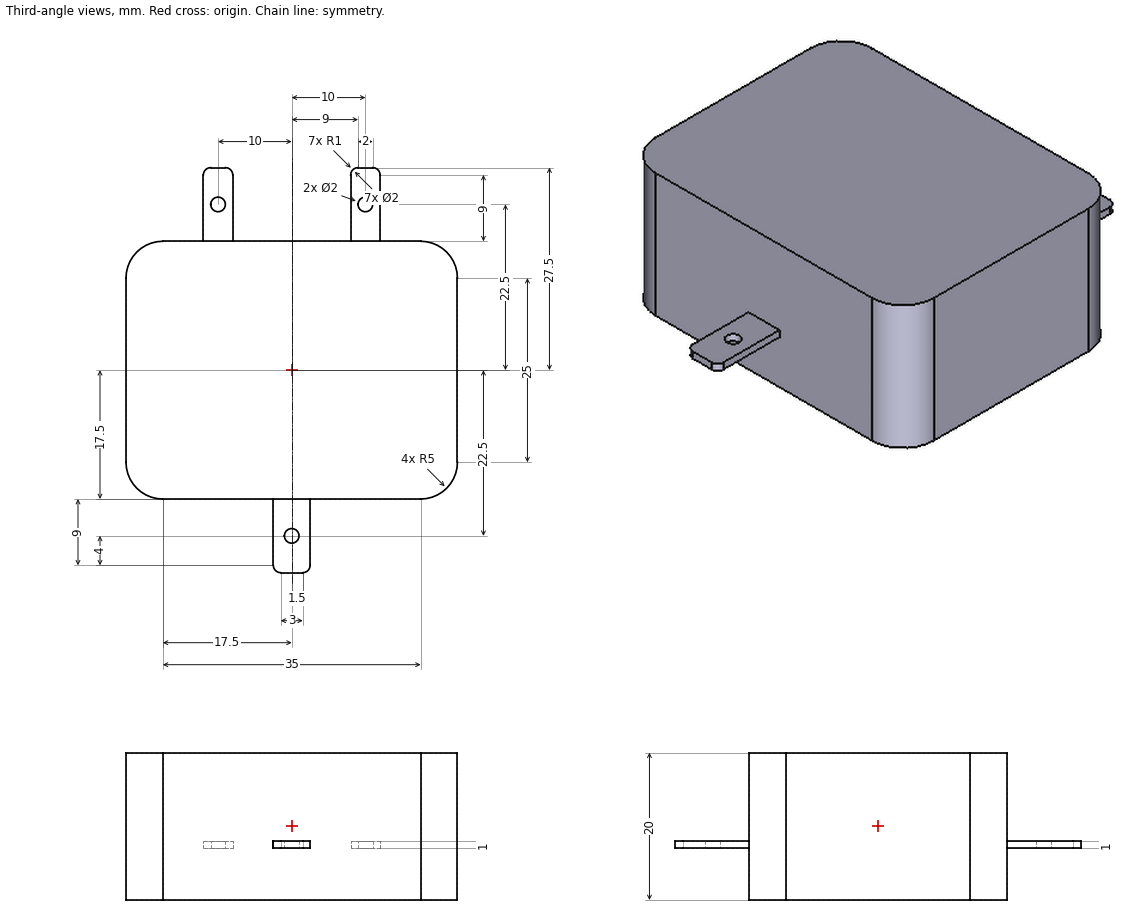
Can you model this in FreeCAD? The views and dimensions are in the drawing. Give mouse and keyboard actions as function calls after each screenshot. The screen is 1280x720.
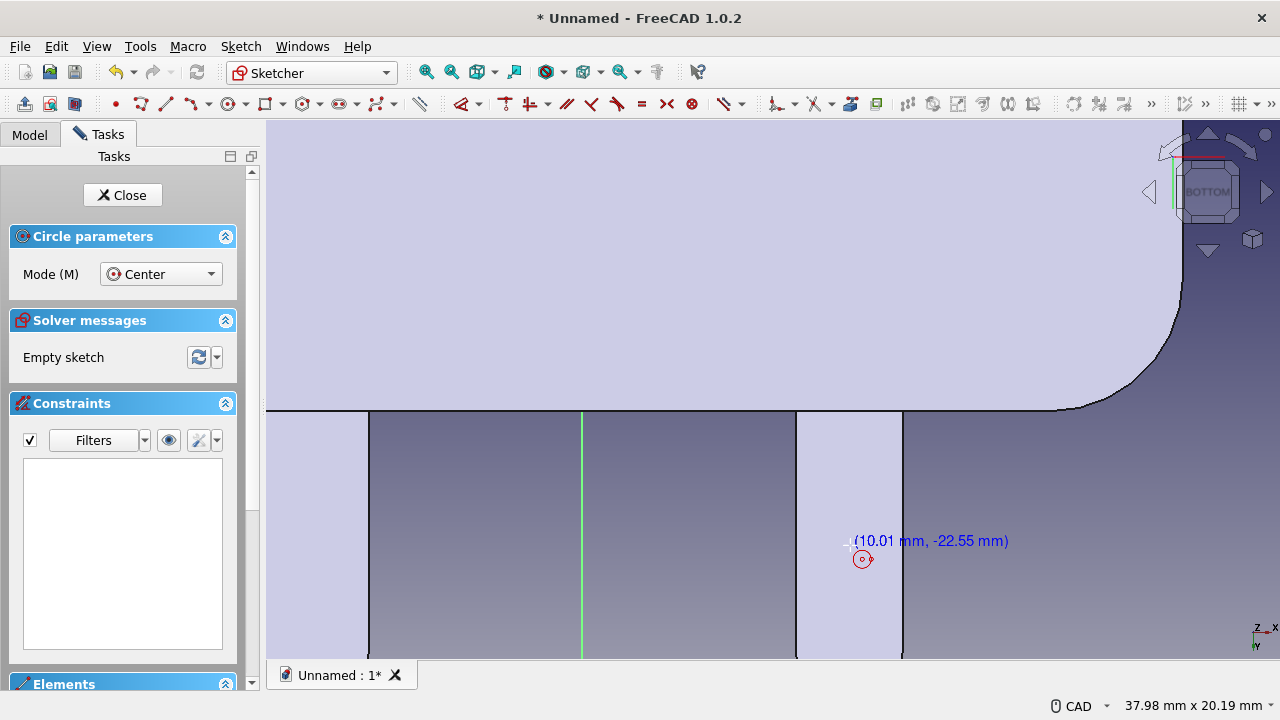
click(849, 545)
click(868, 526)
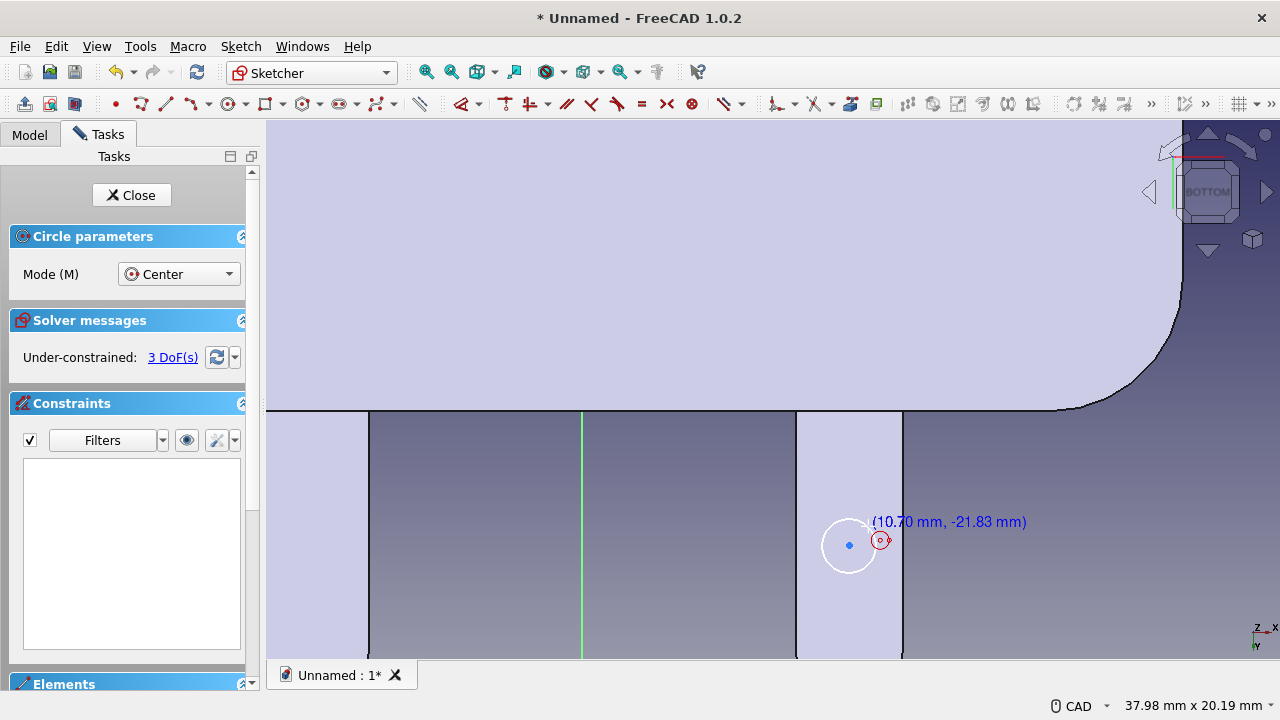
click(315, 545)
click(334, 526)
key(Escape)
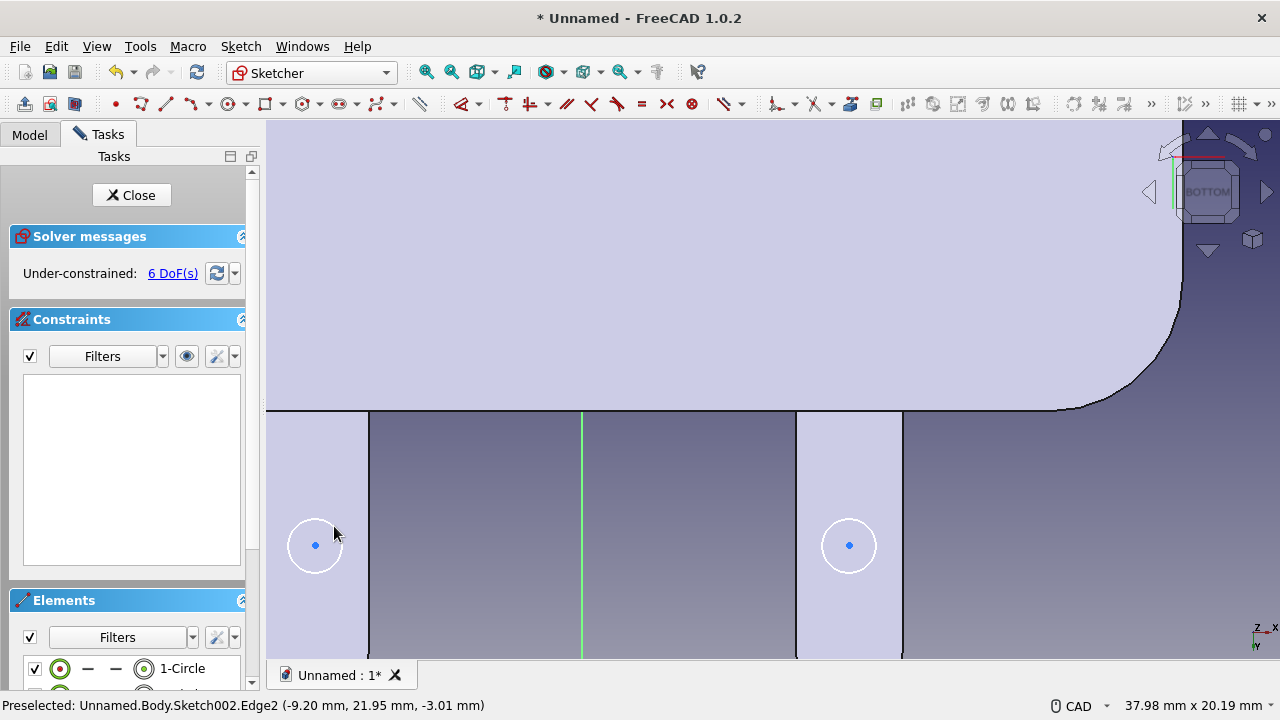
click(868, 527)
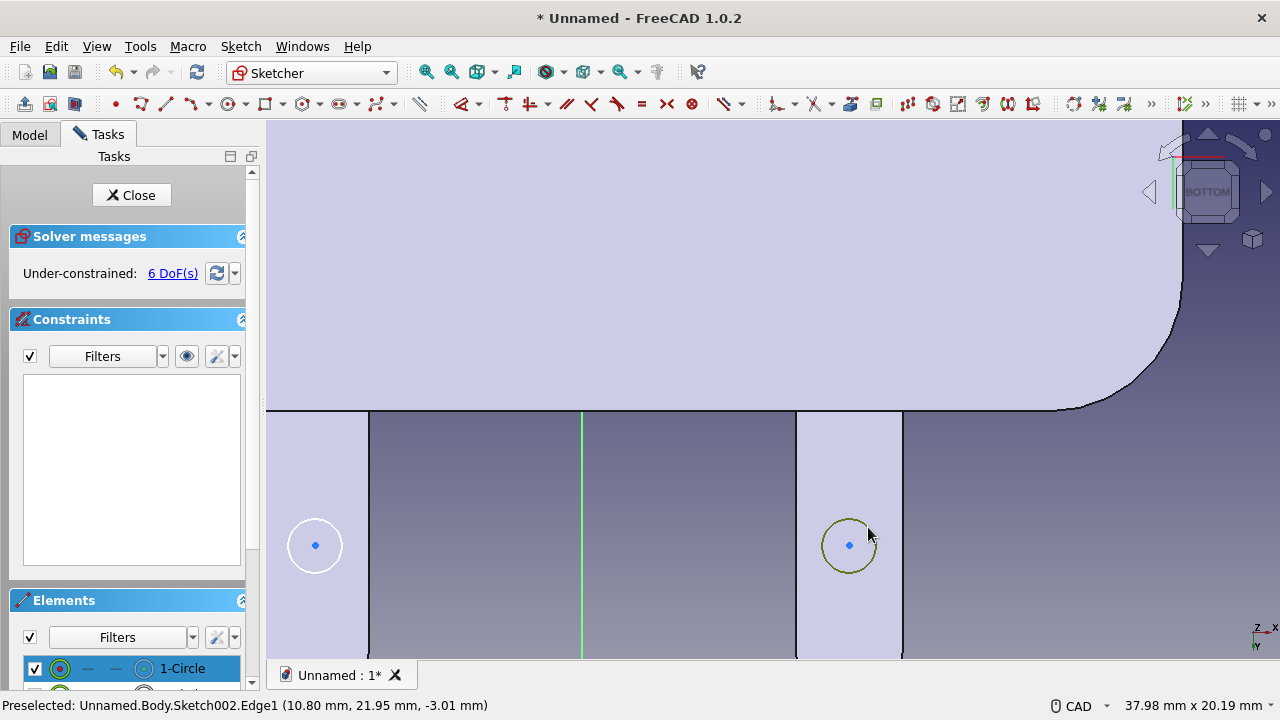
click(334, 527)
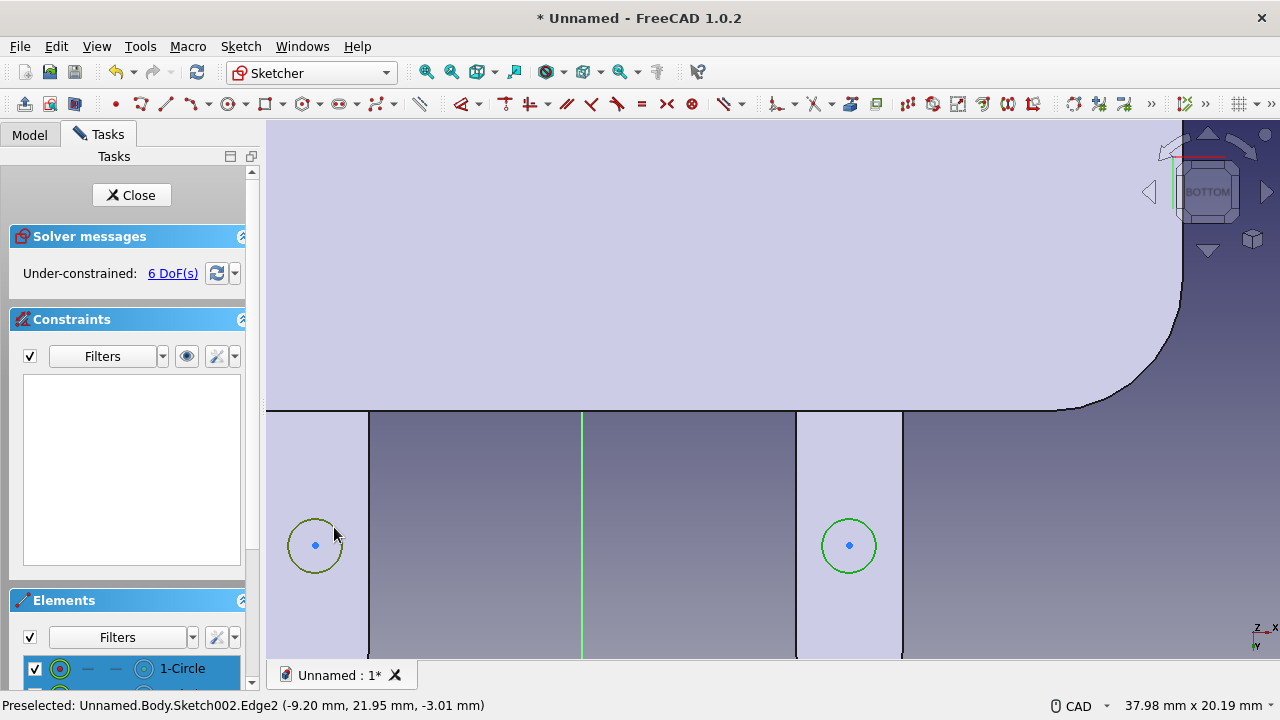
key(e)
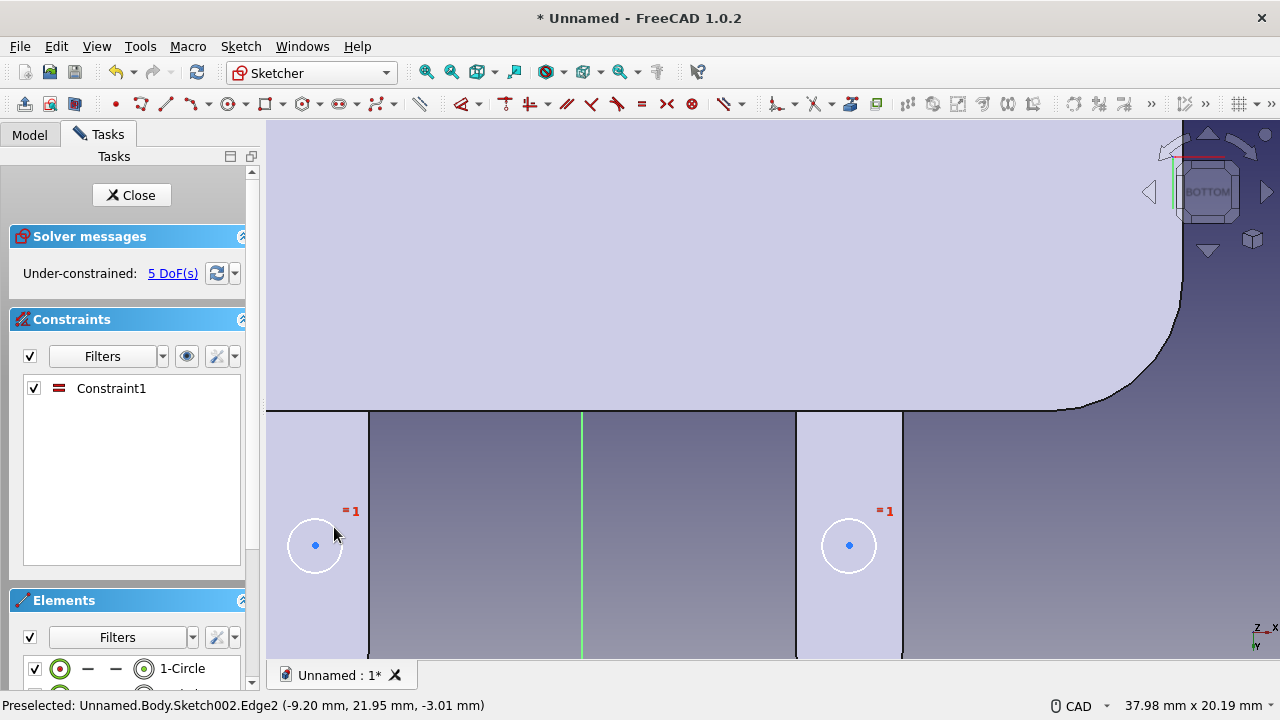
click(849, 546)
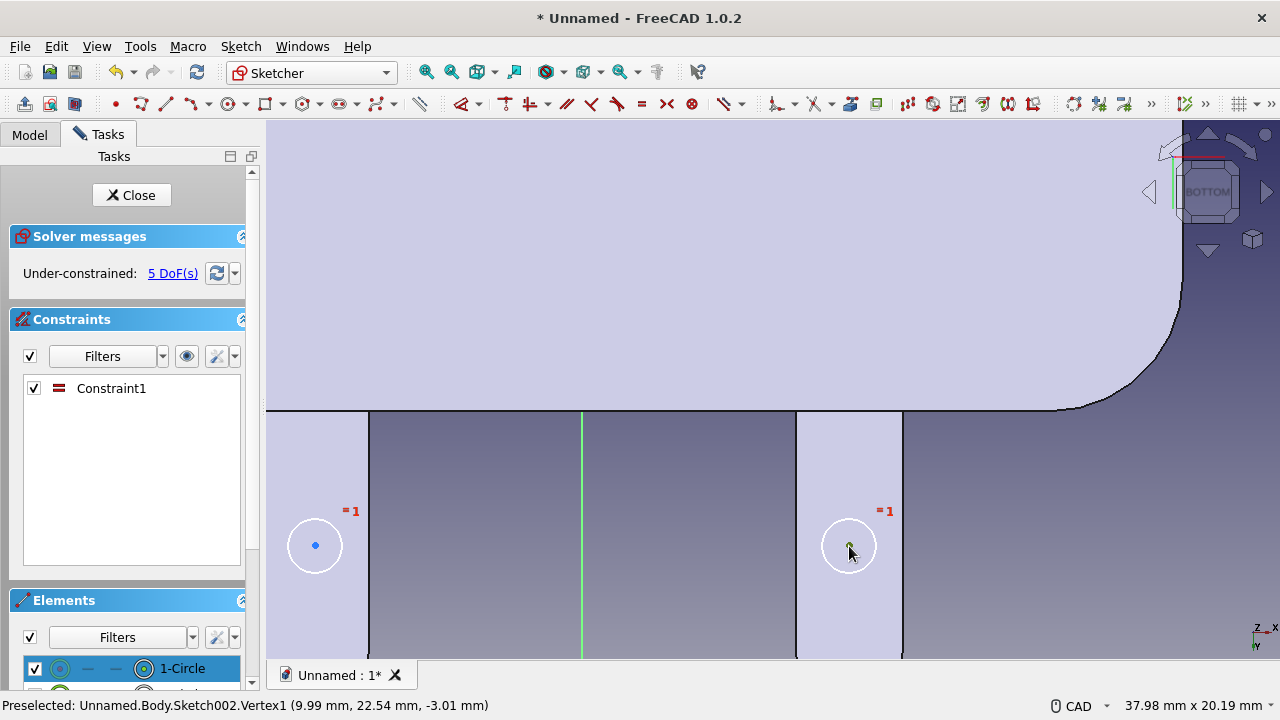
click(315, 546)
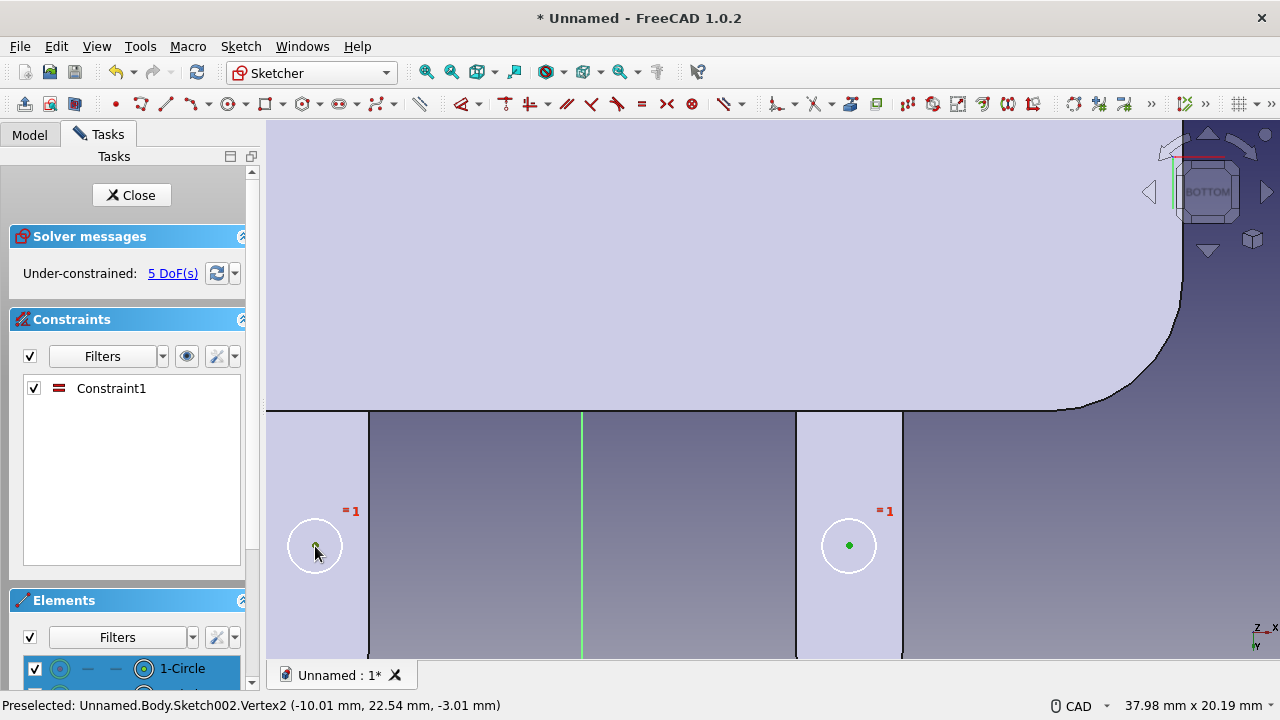
click(548, 104)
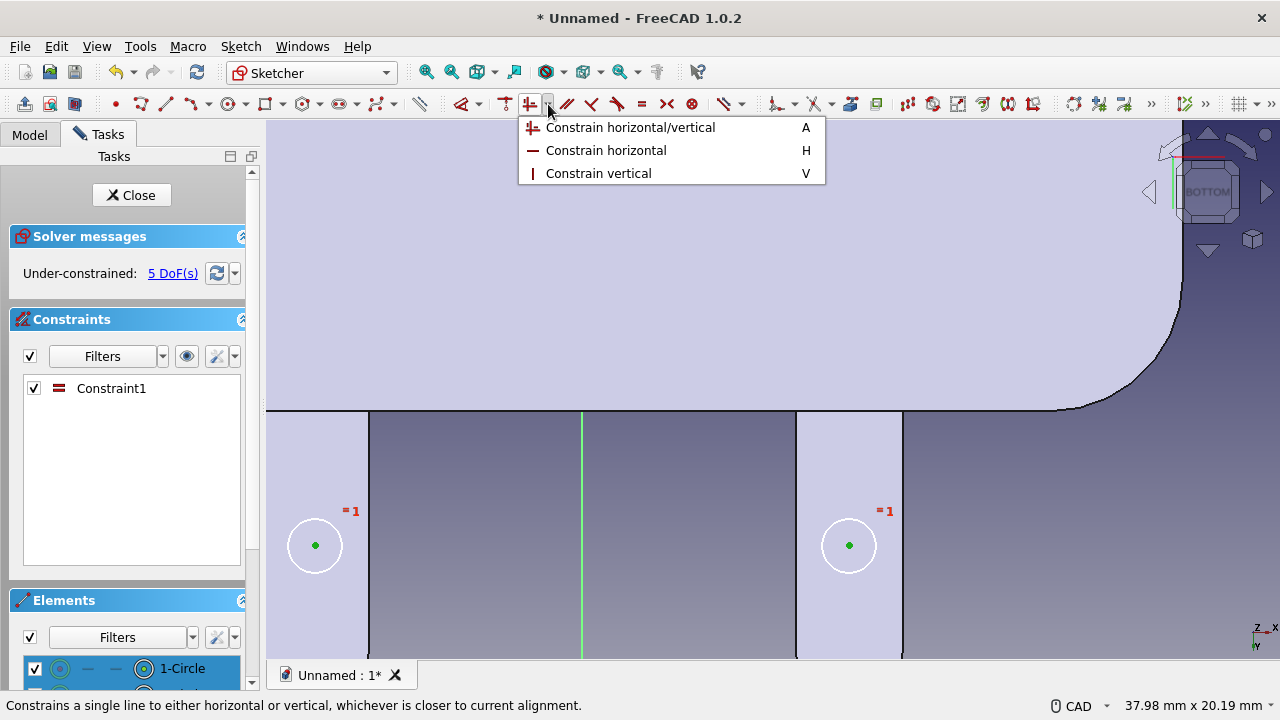
click(672, 150)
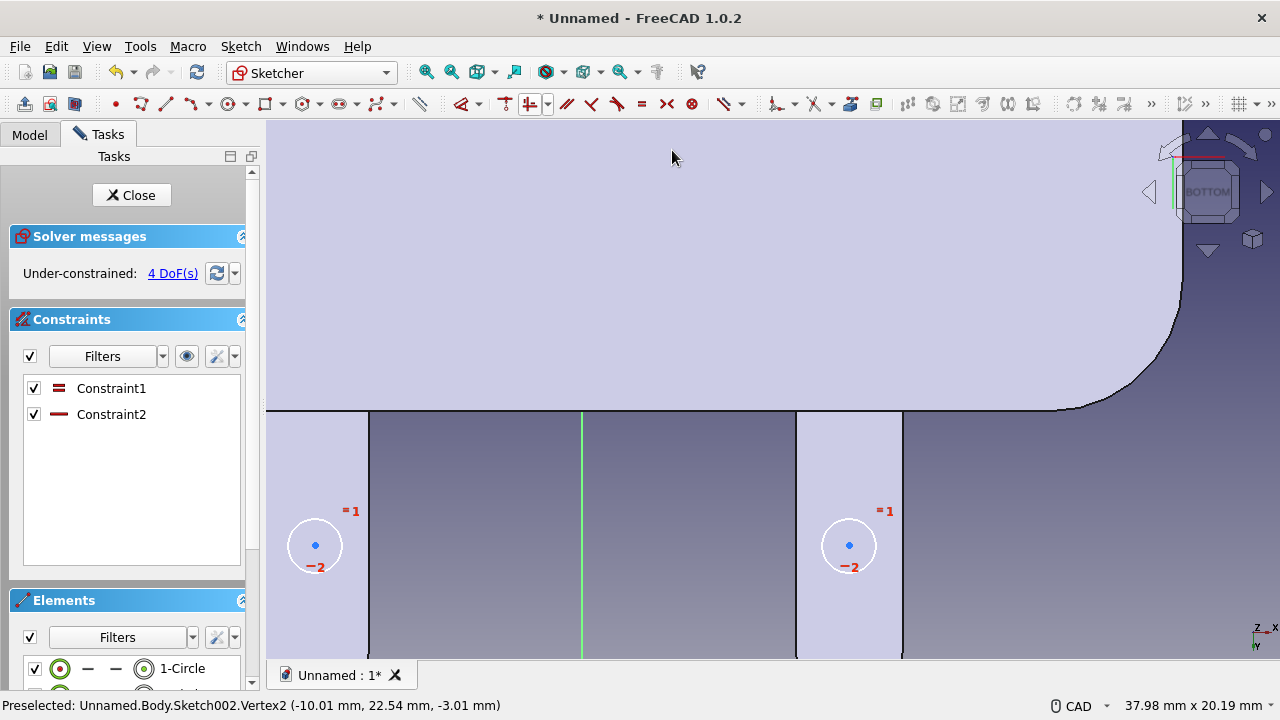
click(460, 104)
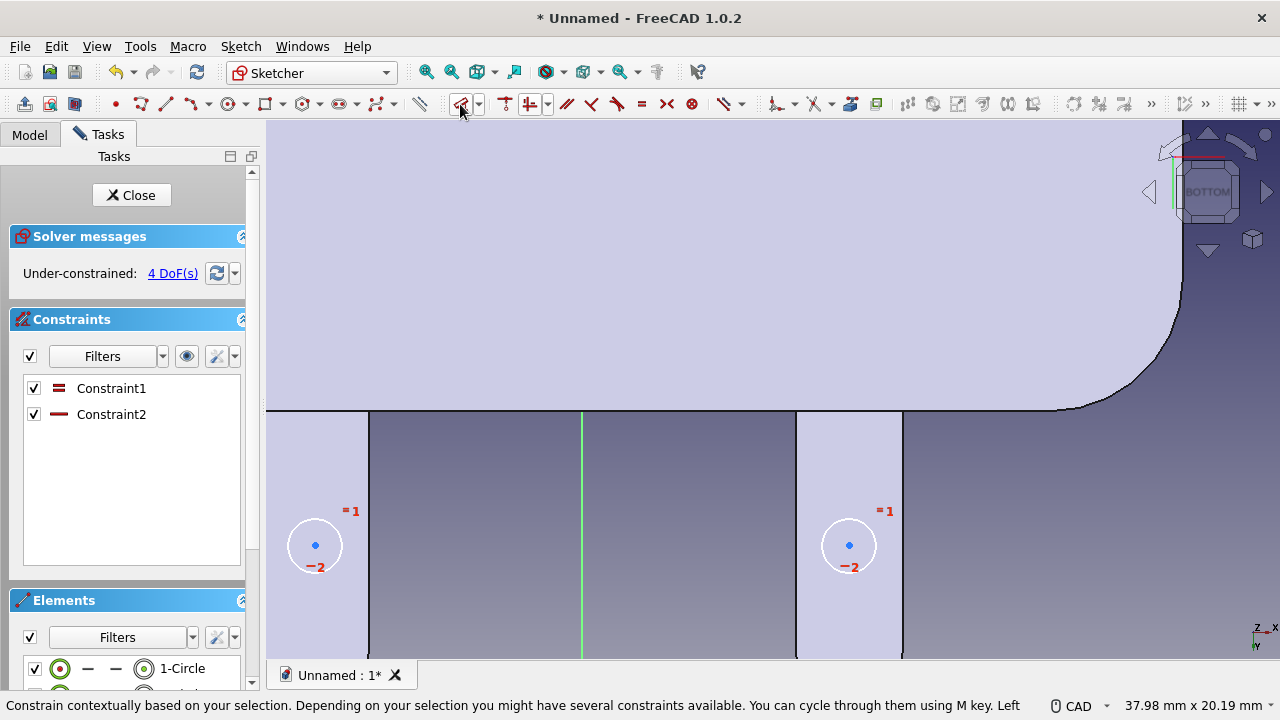
click(868, 527)
click(891, 504)